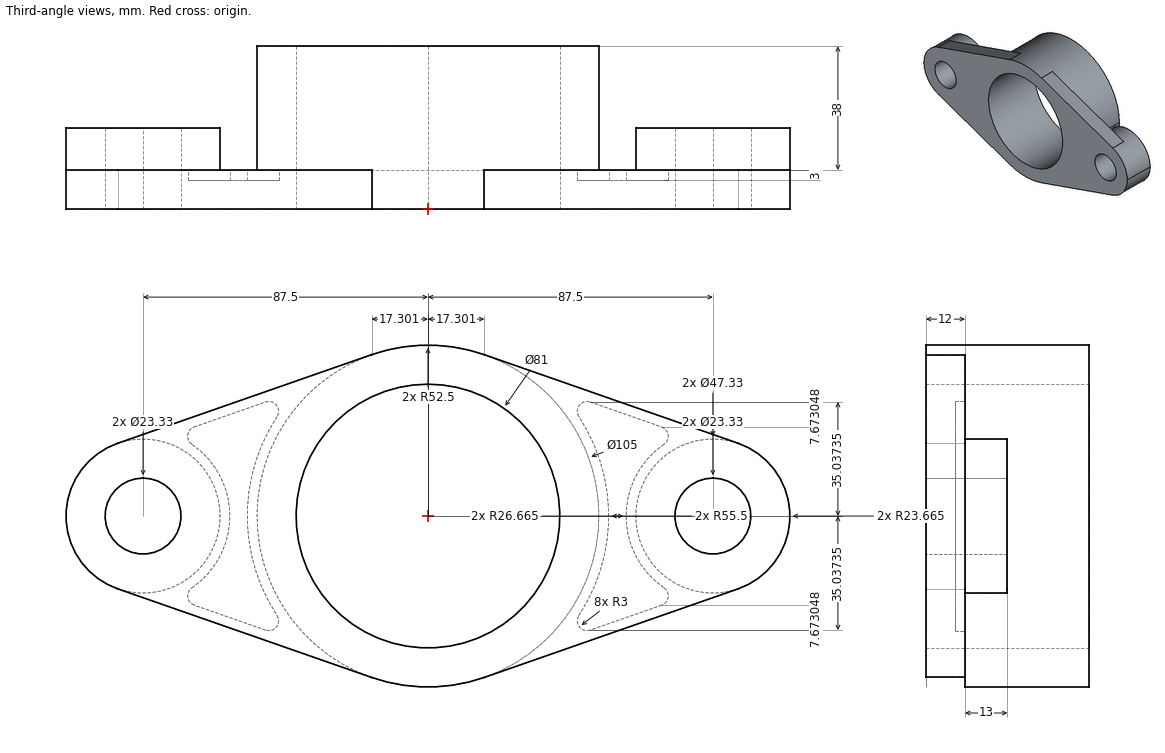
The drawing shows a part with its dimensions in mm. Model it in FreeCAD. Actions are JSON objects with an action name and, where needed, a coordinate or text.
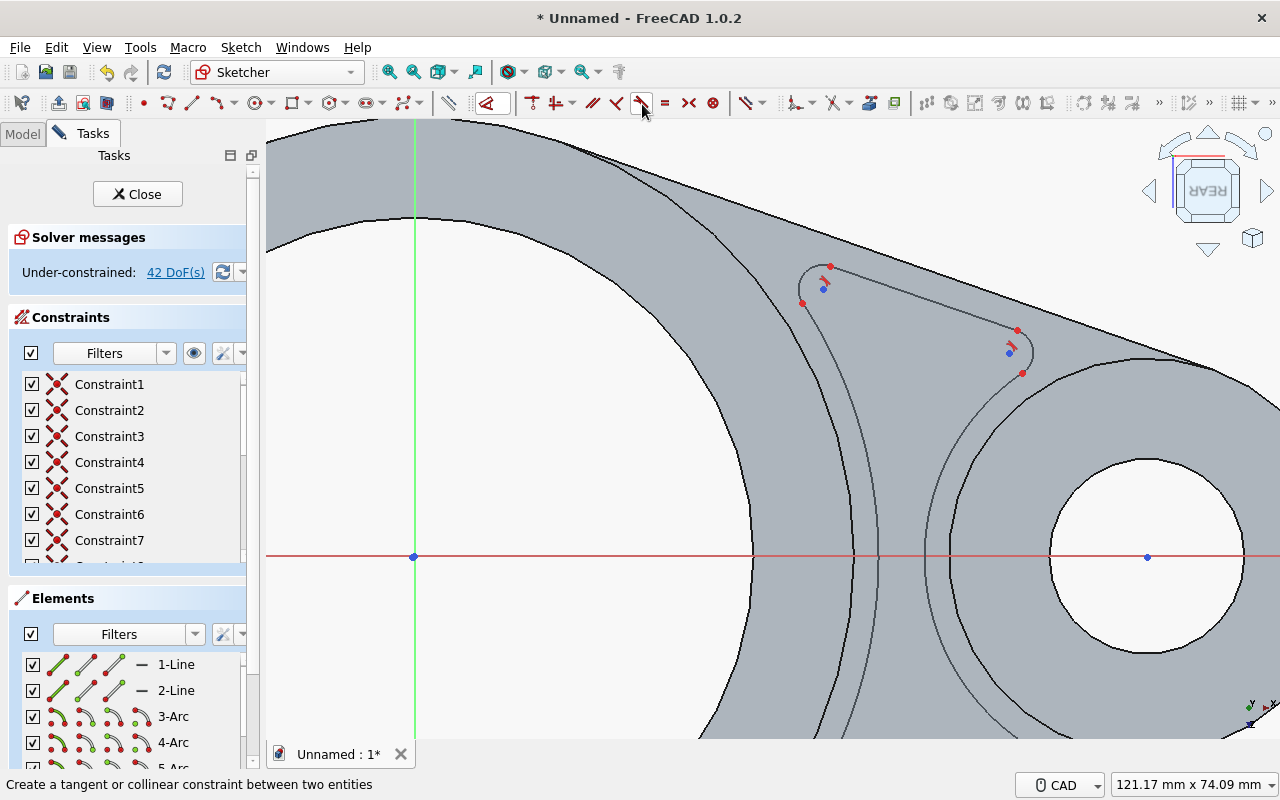
{"action": "scroll", "coordinate": [941, 325], "scroll_direction": "down", "scroll_amount": 4}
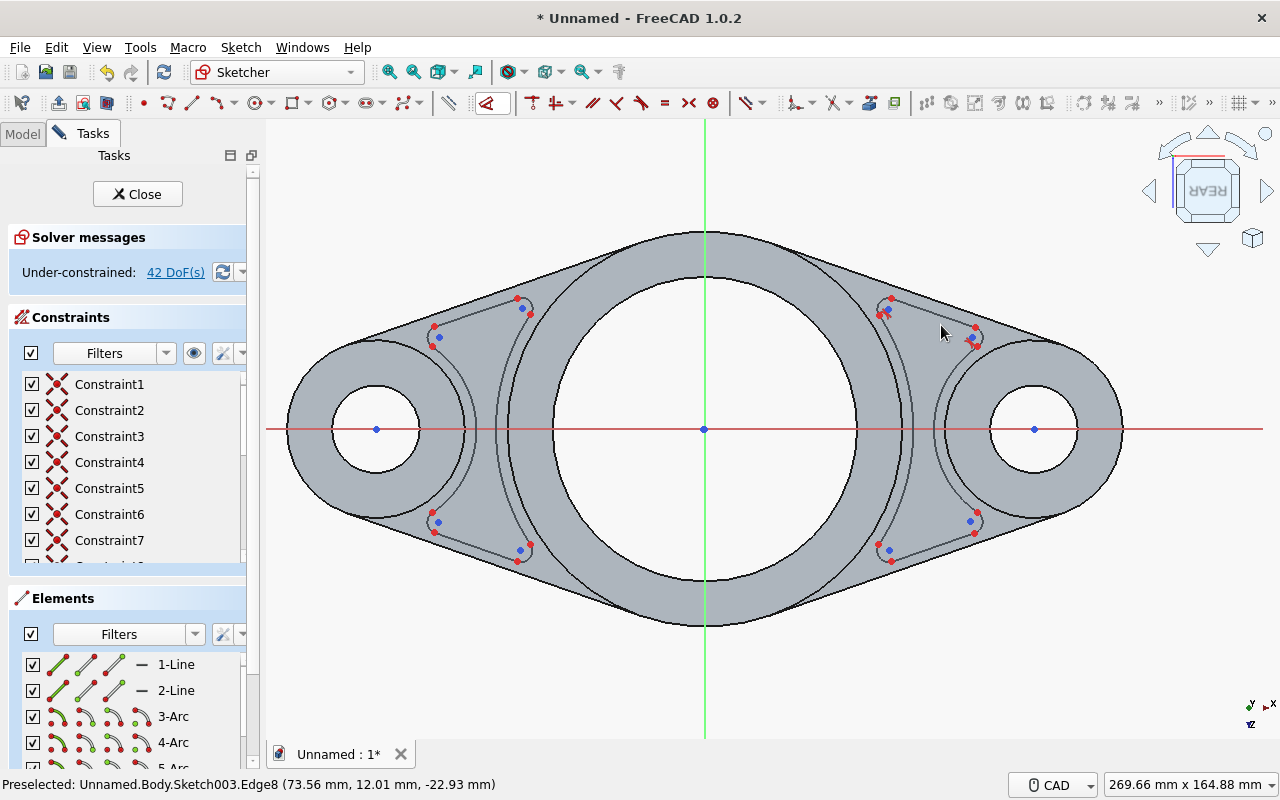
{"action": "left_click", "coordinate": [917, 553]}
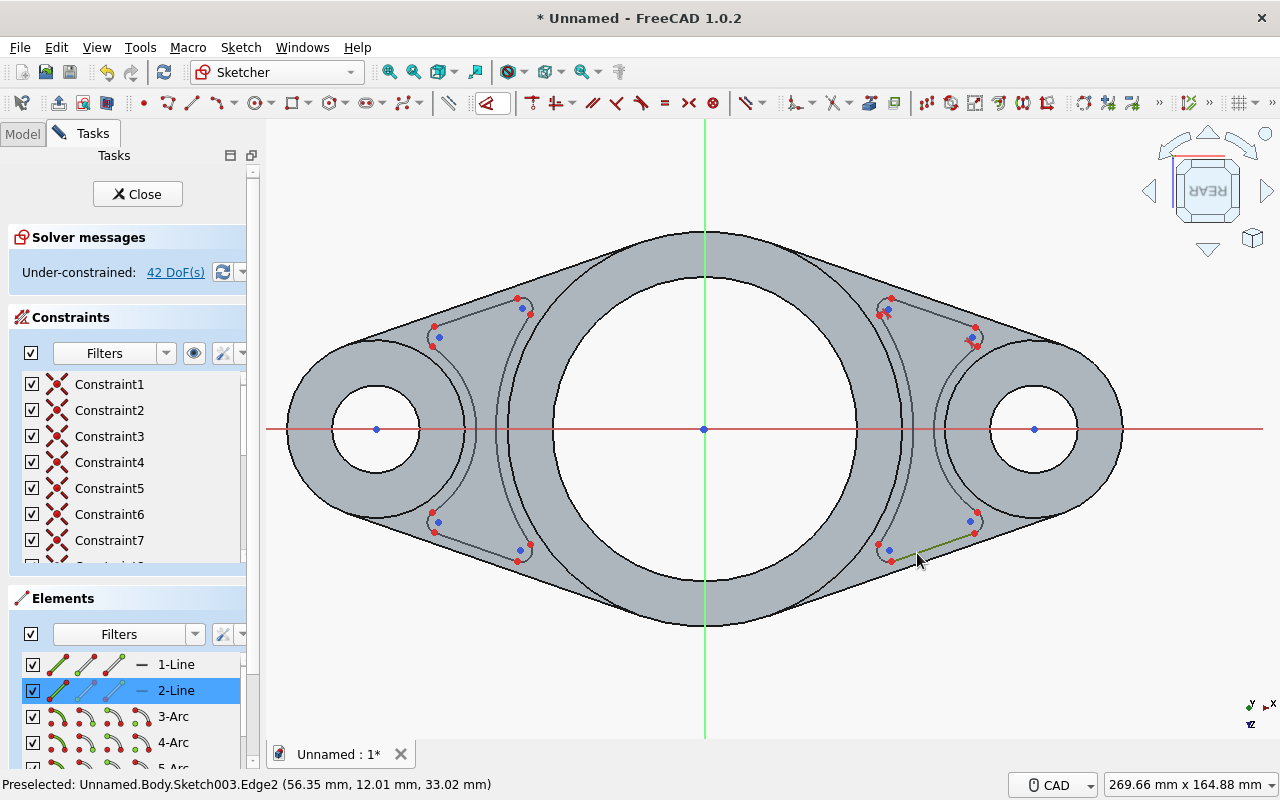
{"action": "left_click", "coordinate": [880, 558]}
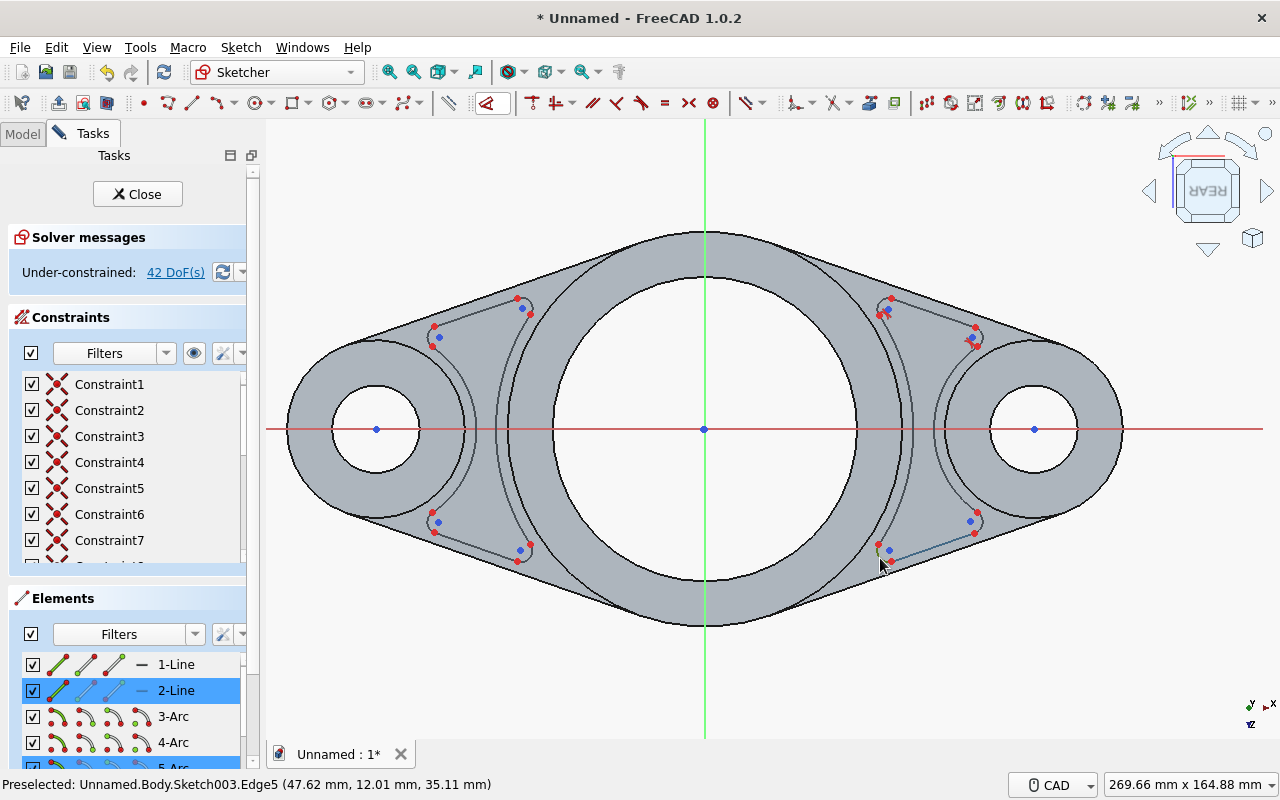
{"action": "left_click", "coordinate": [642, 104]}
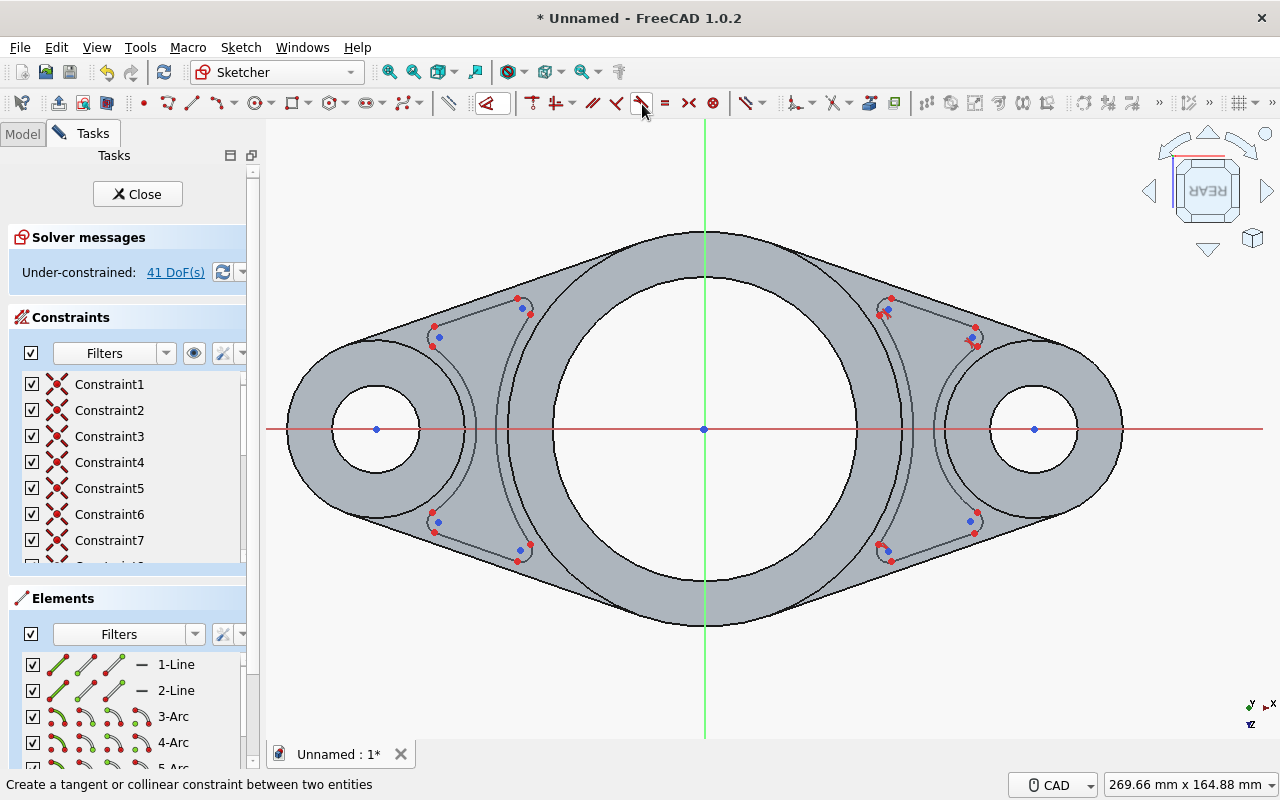
{"action": "left_click", "coordinate": [917, 553]}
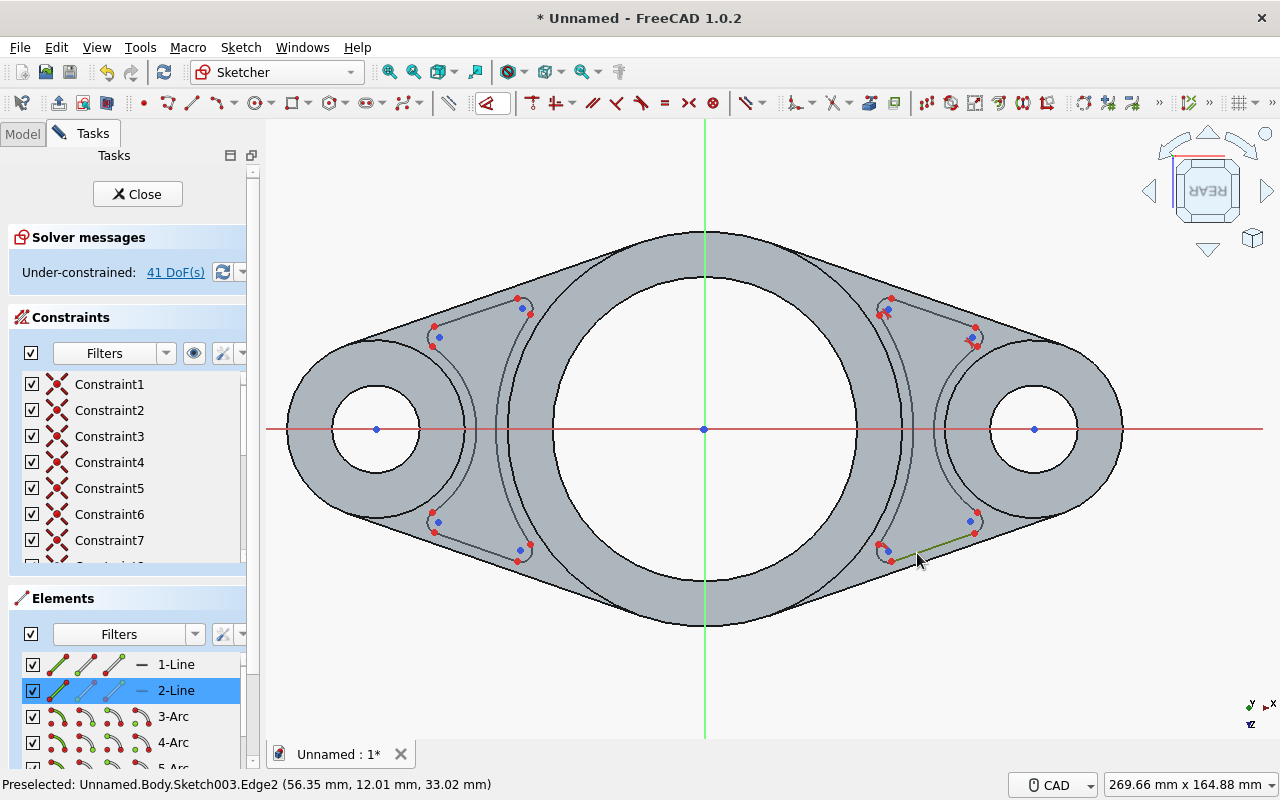
{"action": "left_click", "coordinate": [983, 524]}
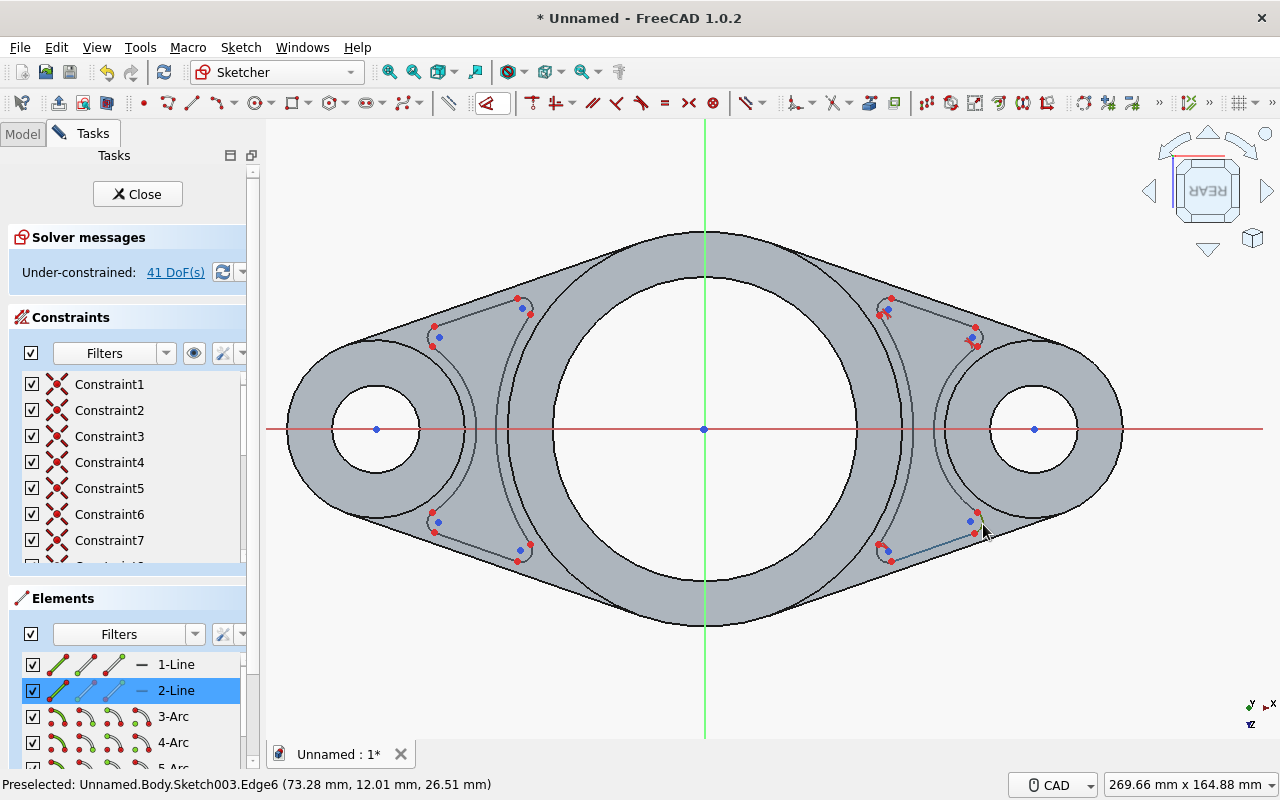
{"action": "left_click", "coordinate": [642, 104]}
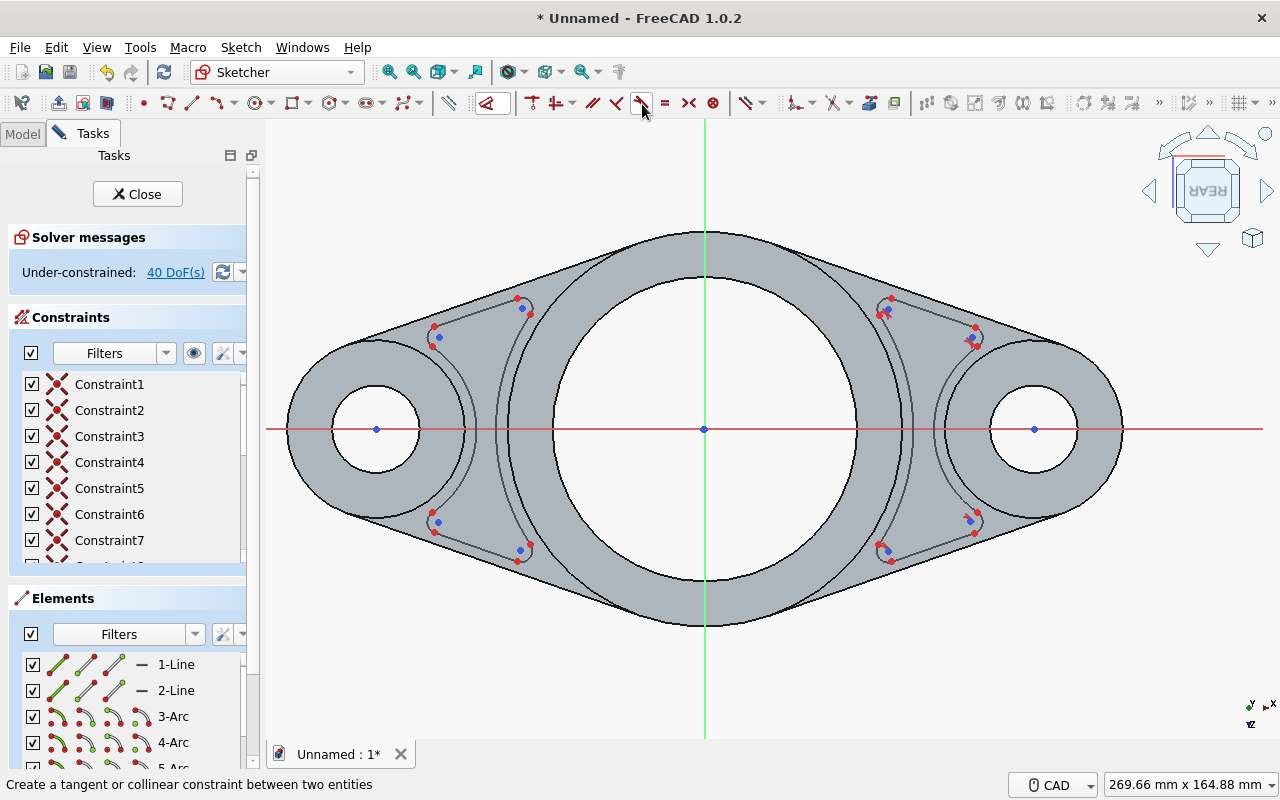
{"action": "scroll", "coordinate": [880, 303], "scroll_direction": "up", "scroll_amount": 2}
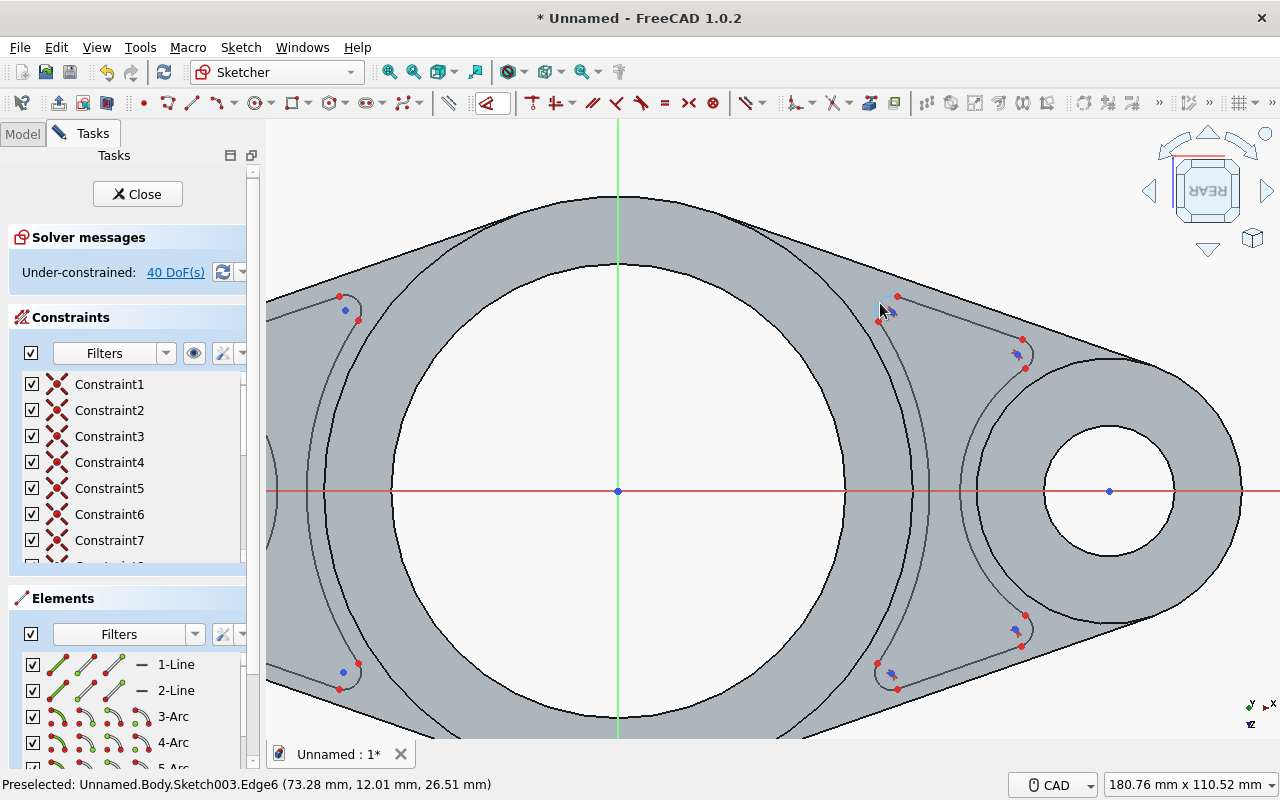
{"action": "left_click", "coordinate": [879, 302]}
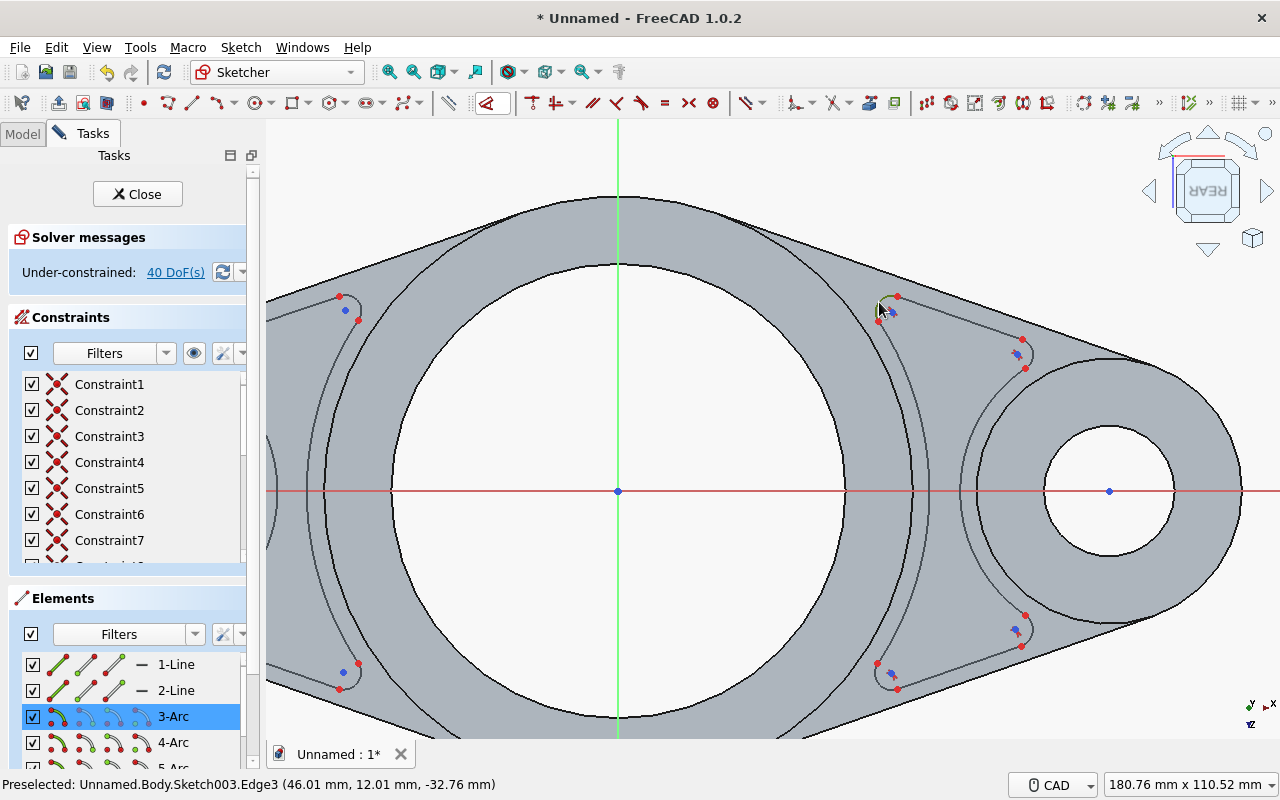
{"action": "left_click", "coordinate": [921, 564]}